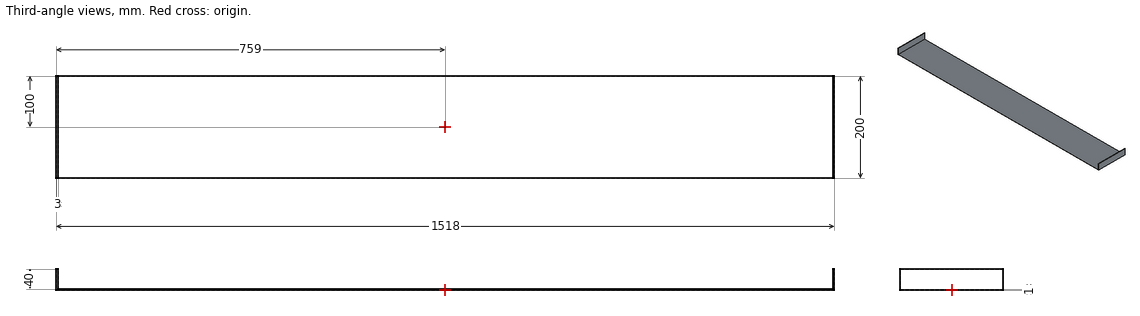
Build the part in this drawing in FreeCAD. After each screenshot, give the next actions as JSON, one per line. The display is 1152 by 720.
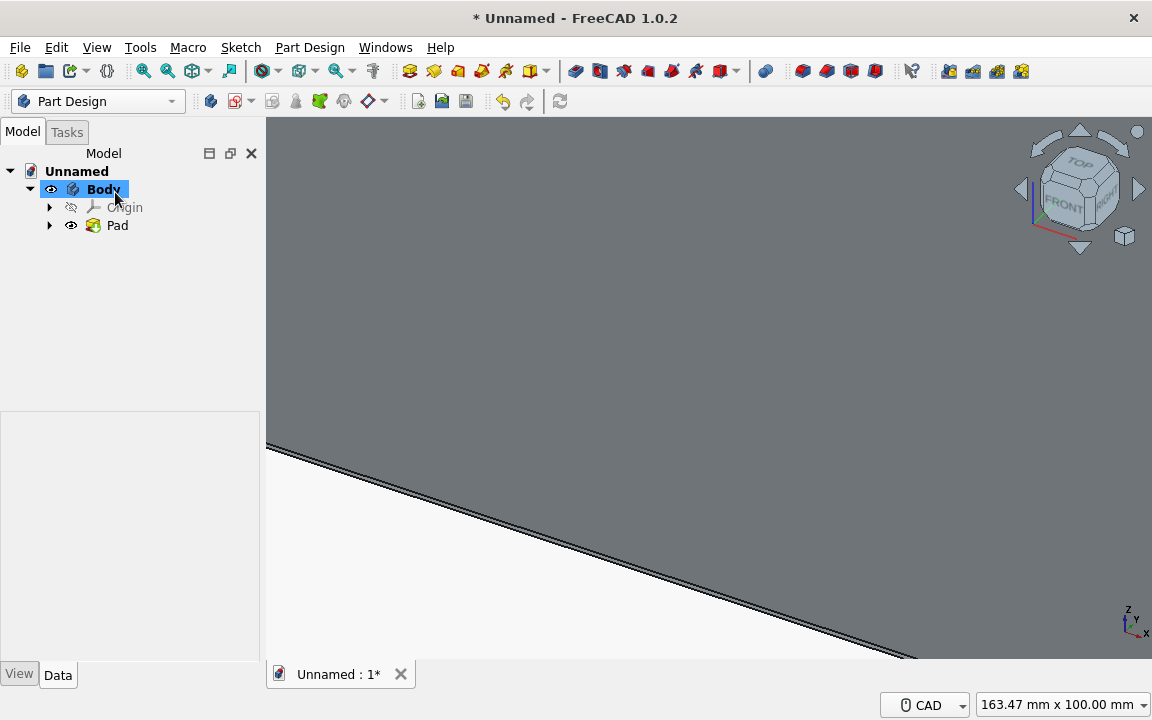
{"action": "left_click", "coordinate": [144, 72]}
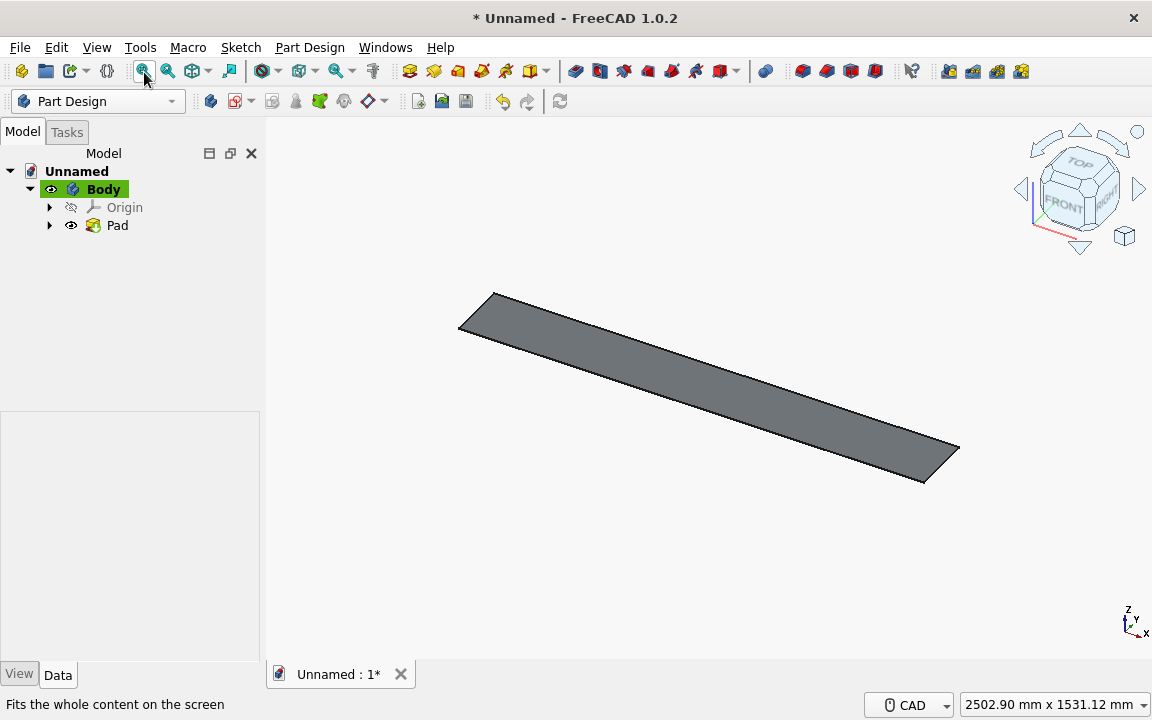
{"action": "left_click", "coordinate": [908, 453]}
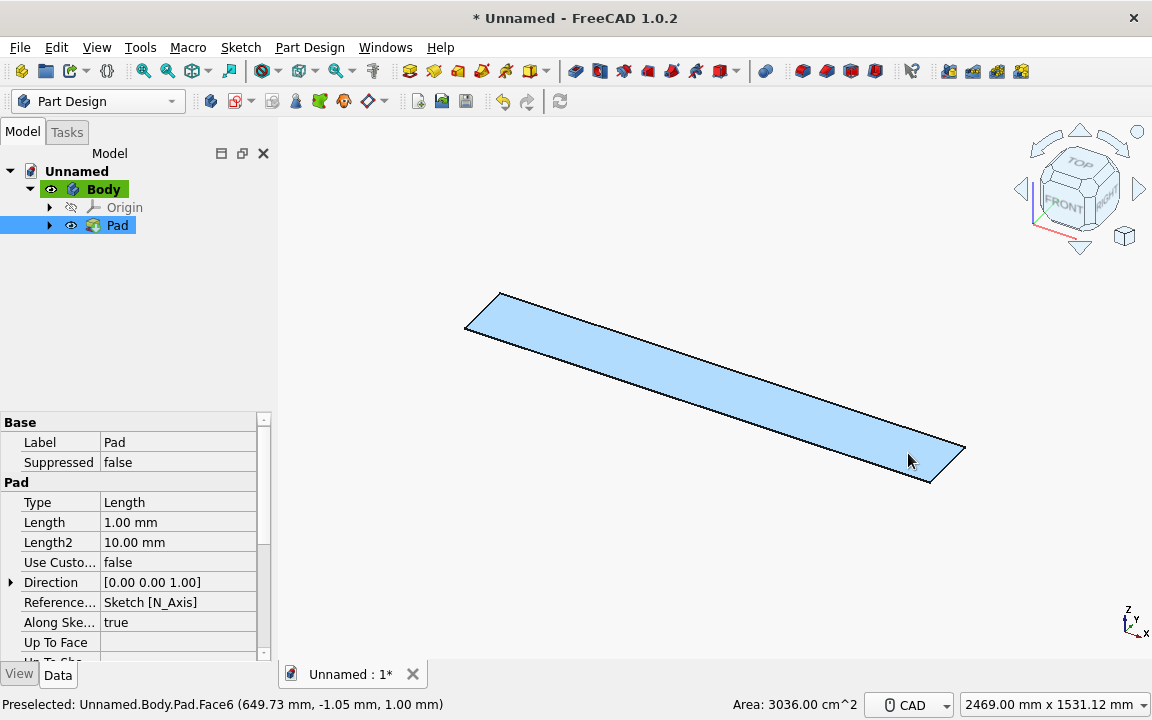
{"action": "left_click", "coordinate": [236, 102]}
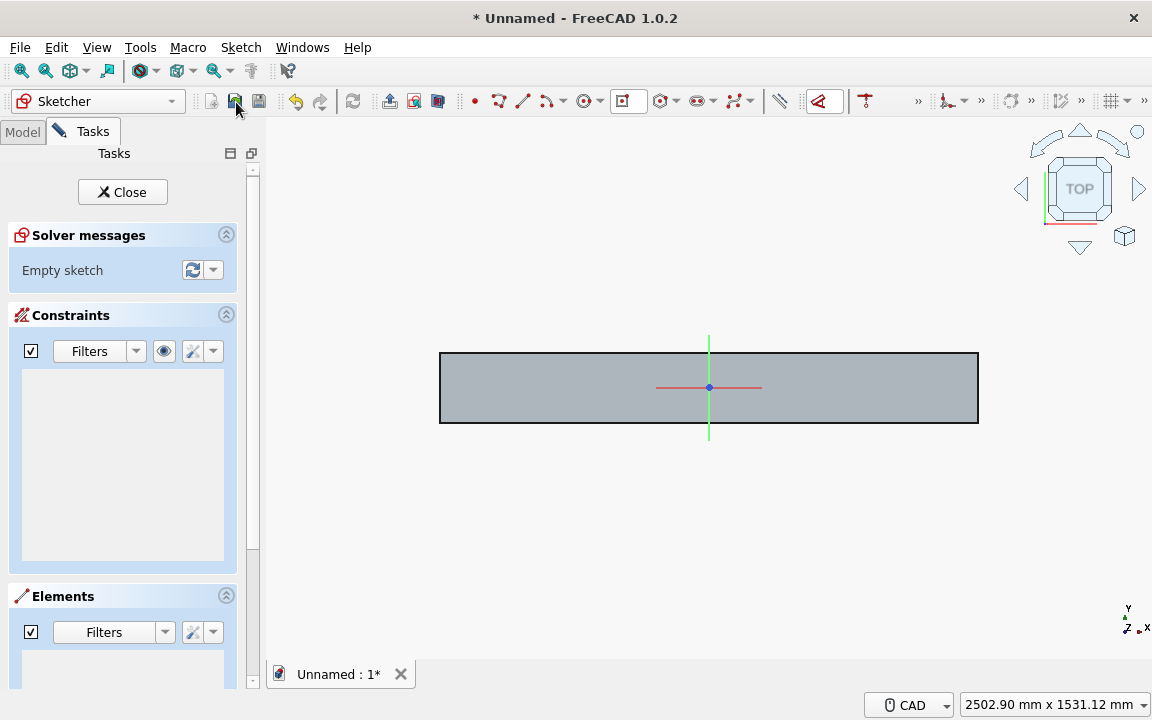
{"action": "scroll", "coordinate": [390, 388], "scroll_direction": "up", "scroll_amount": 8}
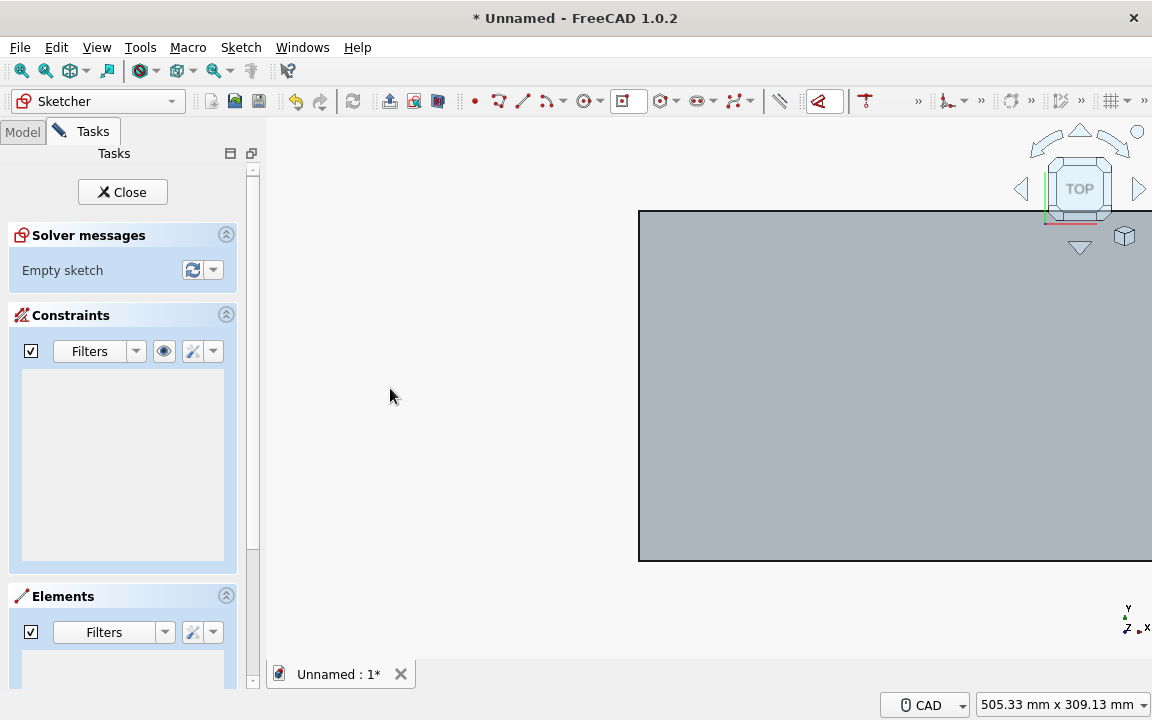
{"action": "key", "text": "g r"}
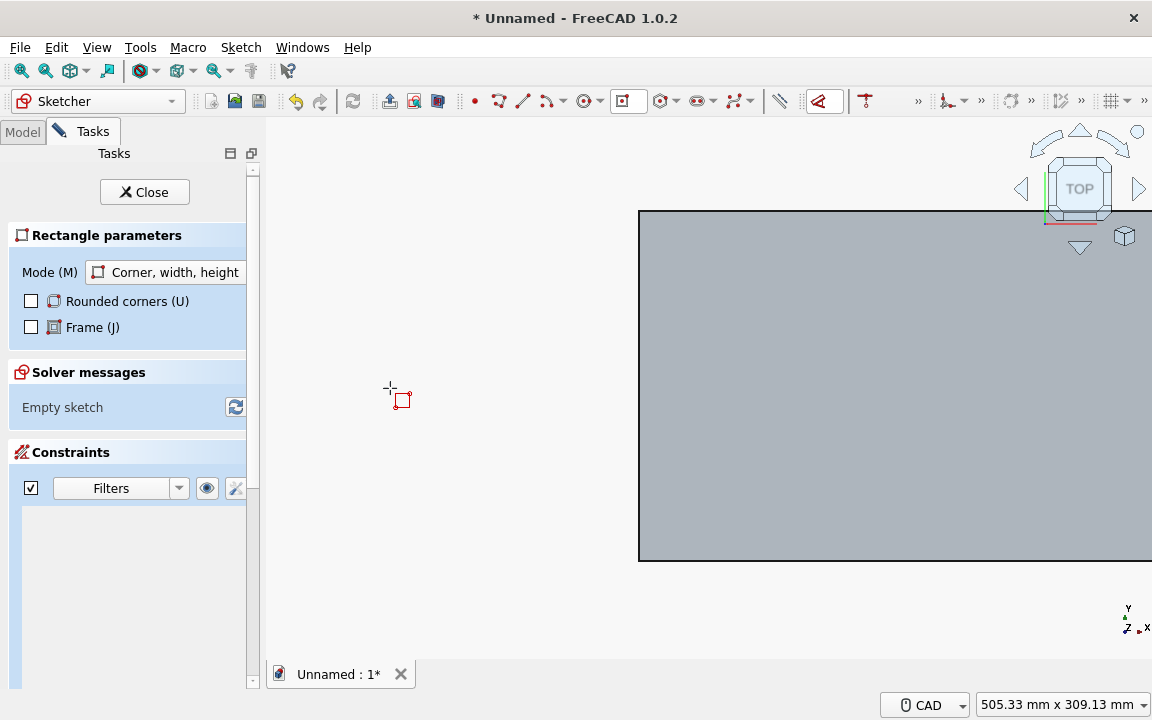
{"action": "scroll", "coordinate": [639, 211], "scroll_direction": "up", "scroll_amount": 6}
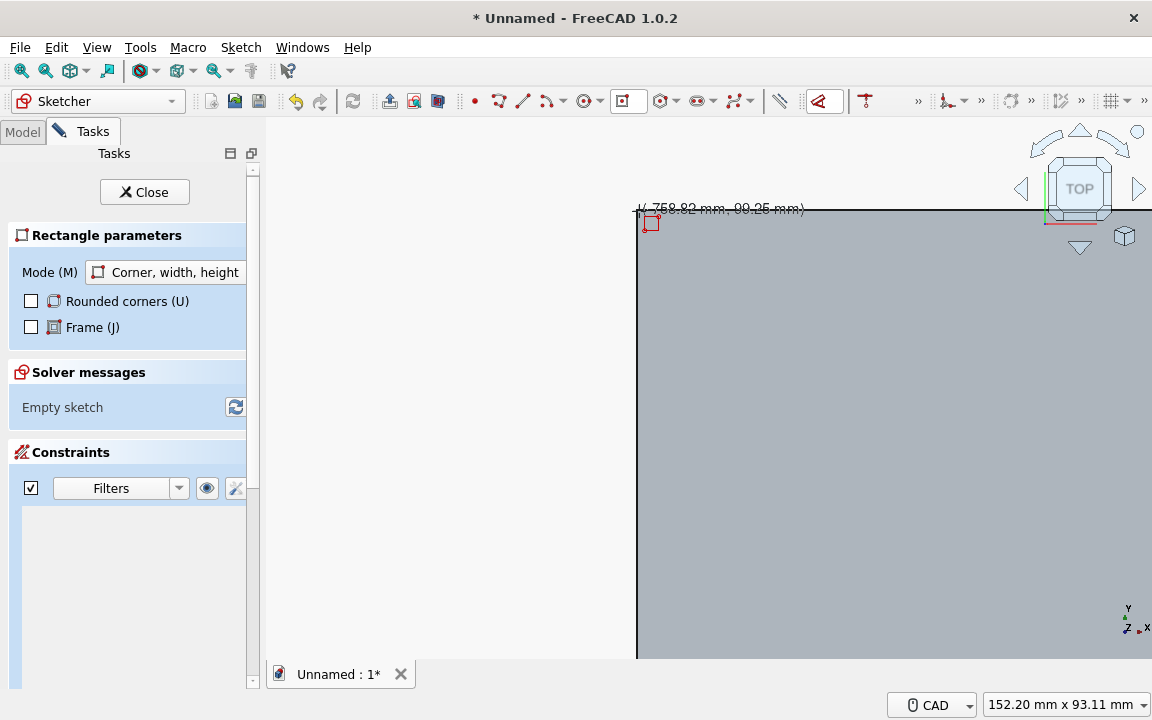
{"action": "left_click", "coordinate": [637, 210]}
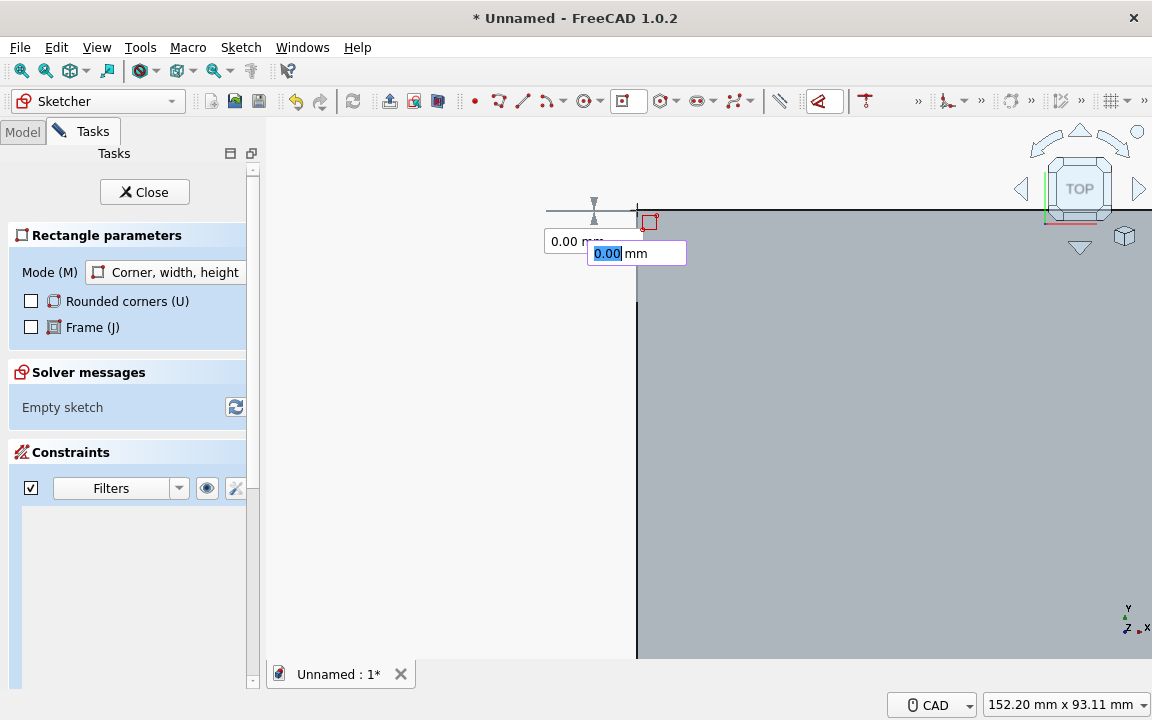
{"action": "scroll", "coordinate": [638, 214], "scroll_direction": "down", "scroll_amount": 6}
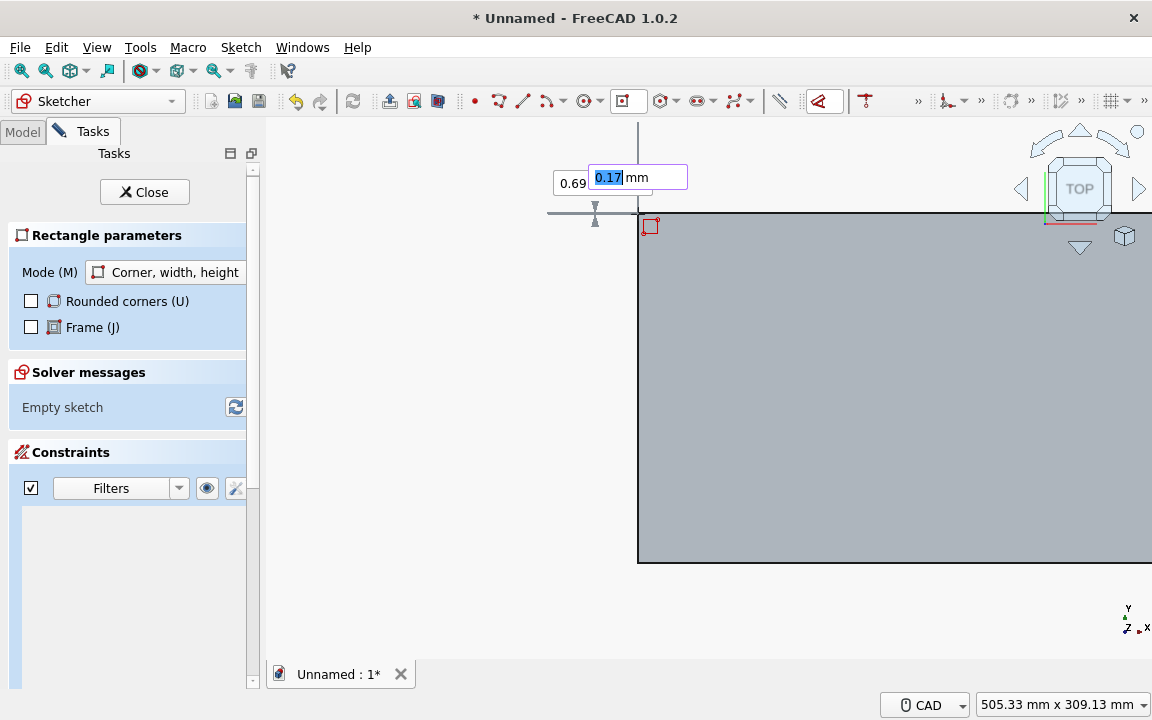
{"action": "left_click", "coordinate": [643, 563]}
{"action": "key", "text": "Escape"}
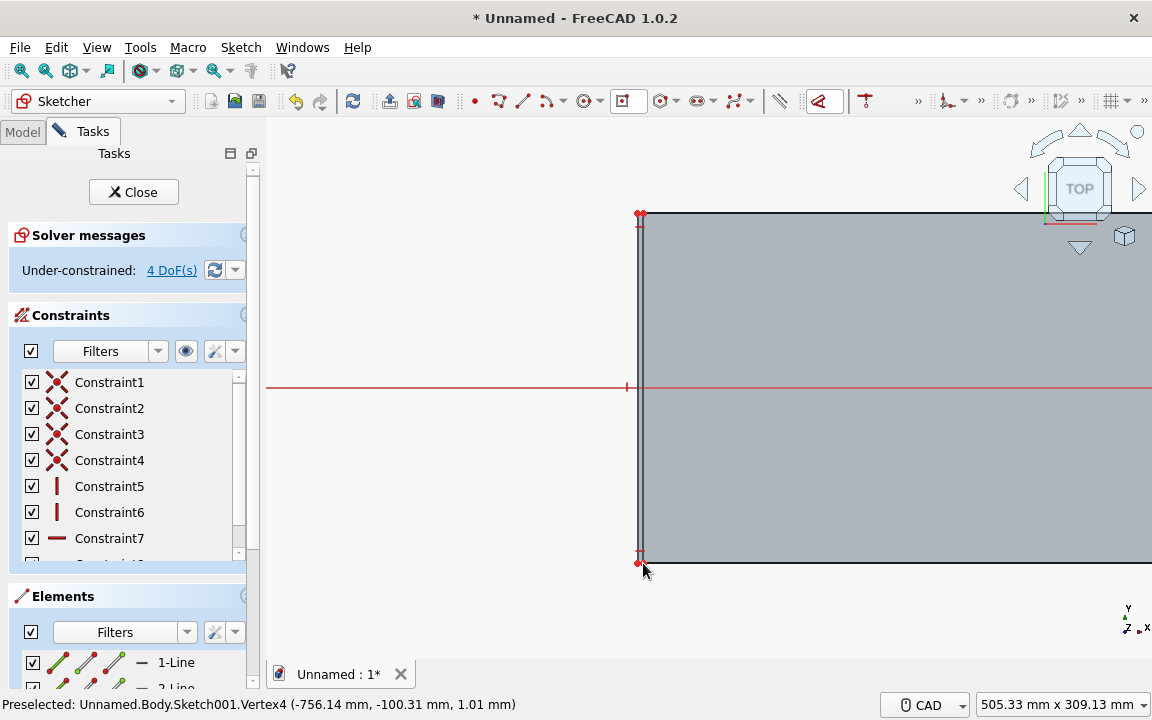
{"action": "left_click", "coordinate": [818, 102]}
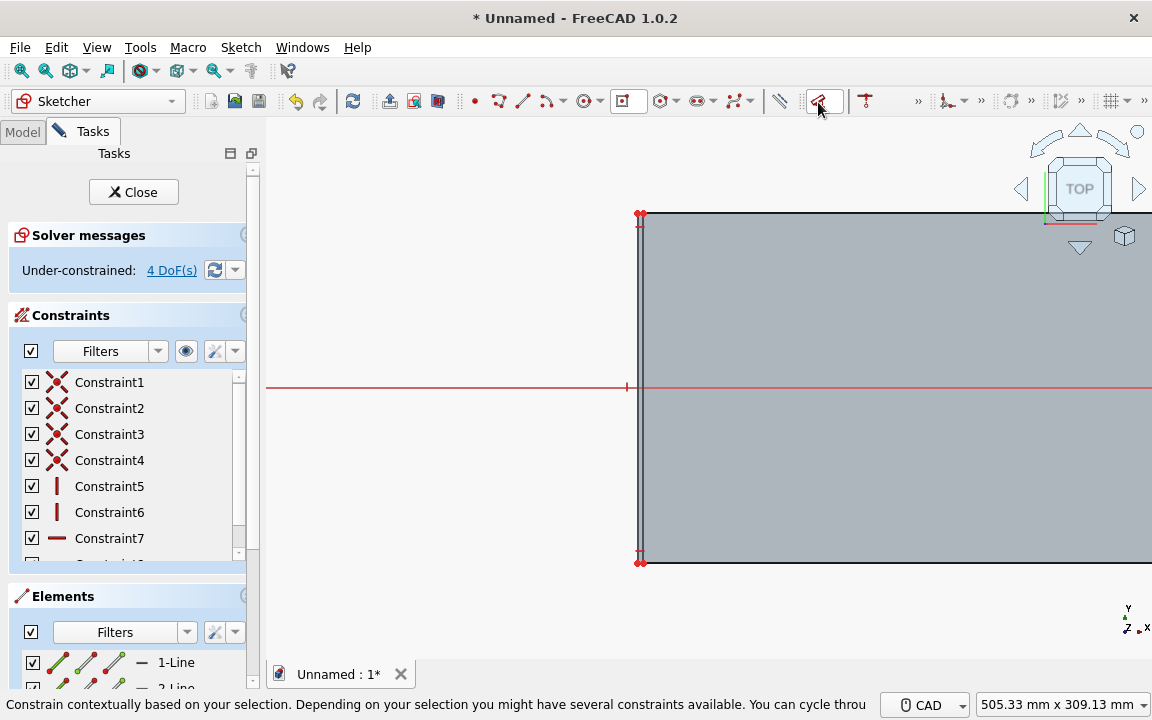
{"action": "scroll", "coordinate": [640, 564], "scroll_direction": "up", "scroll_amount": 11}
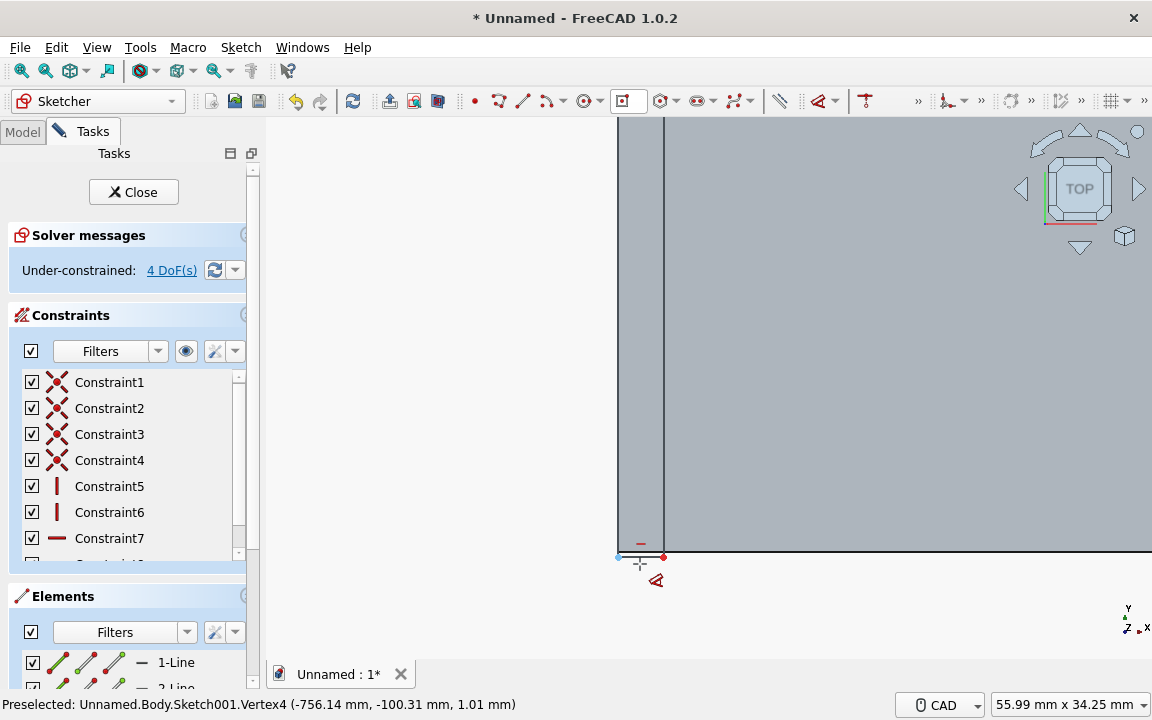
{"action": "left_click", "coordinate": [641, 557]}
{"action": "left_click", "coordinate": [641, 591]}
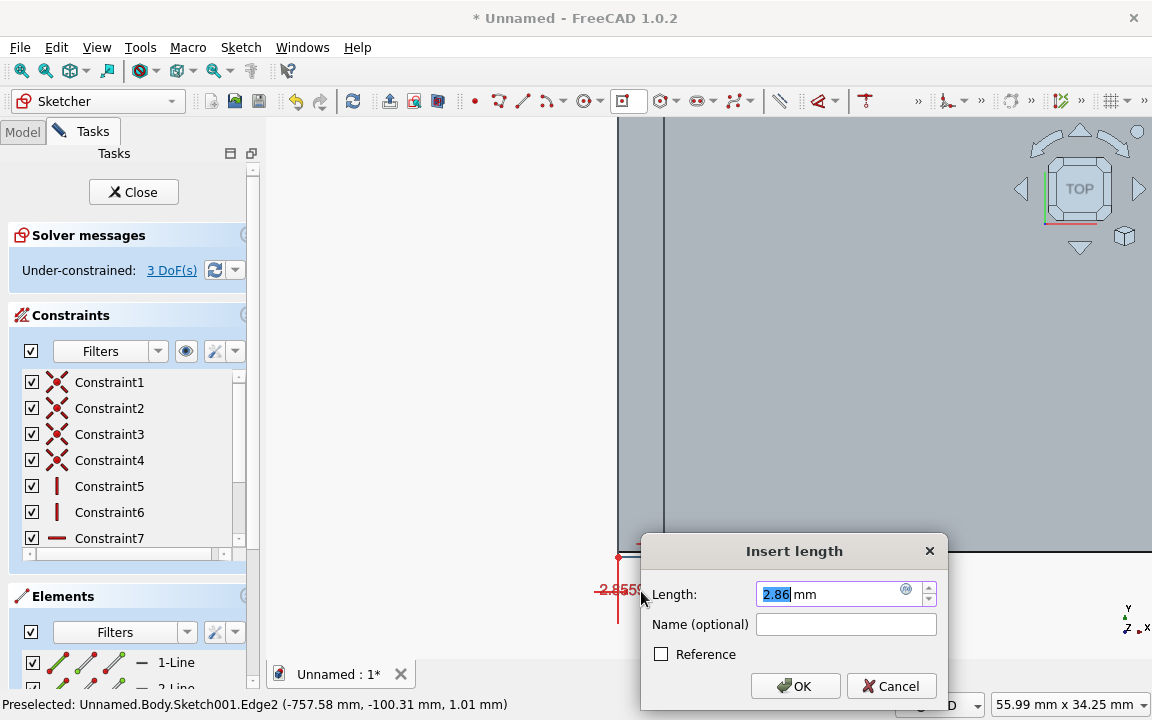
{"action": "type", "text": "3"}
{"action": "key", "text": "Return"}